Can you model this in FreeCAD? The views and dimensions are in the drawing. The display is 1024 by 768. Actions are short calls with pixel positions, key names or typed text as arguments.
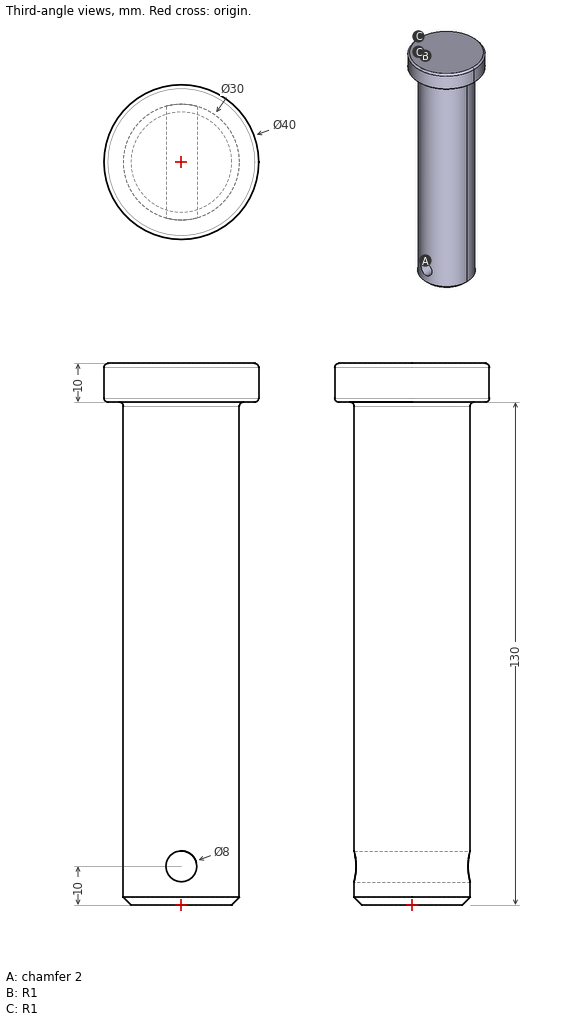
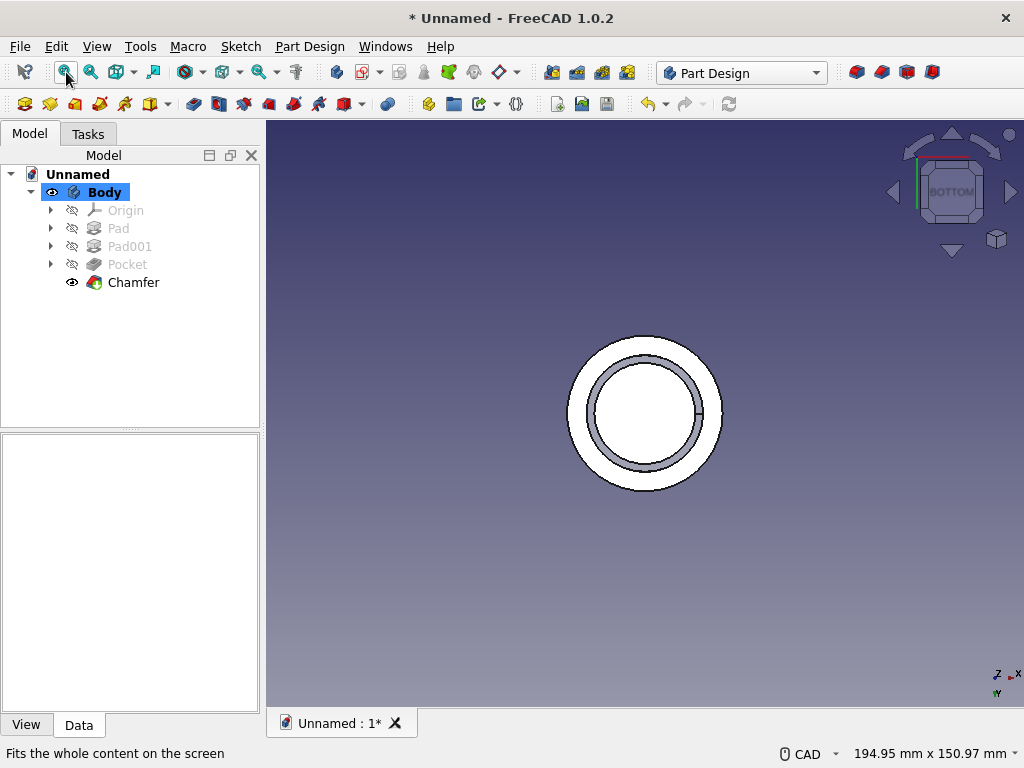
key(4)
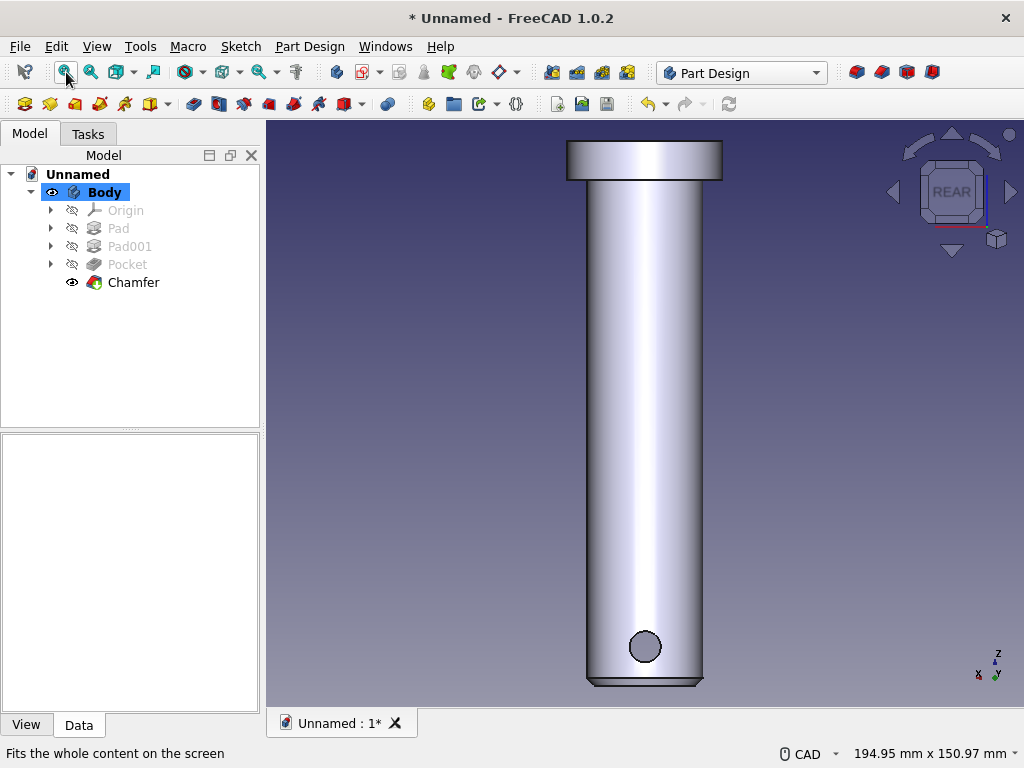
key(6)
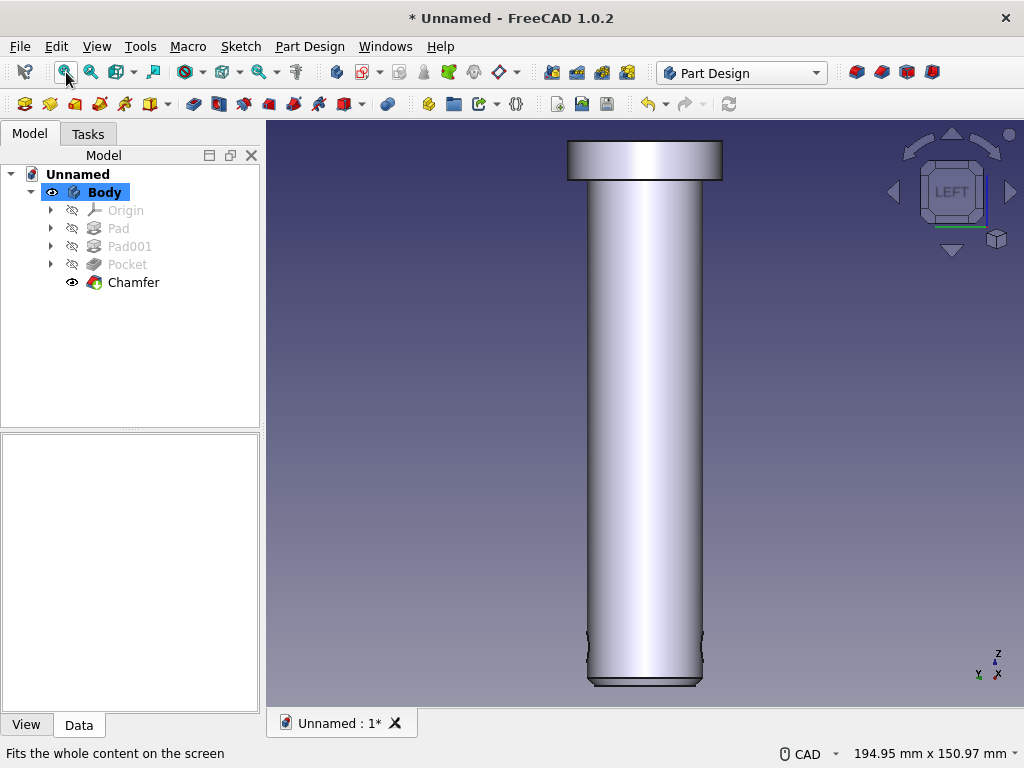
key(v)
key(3)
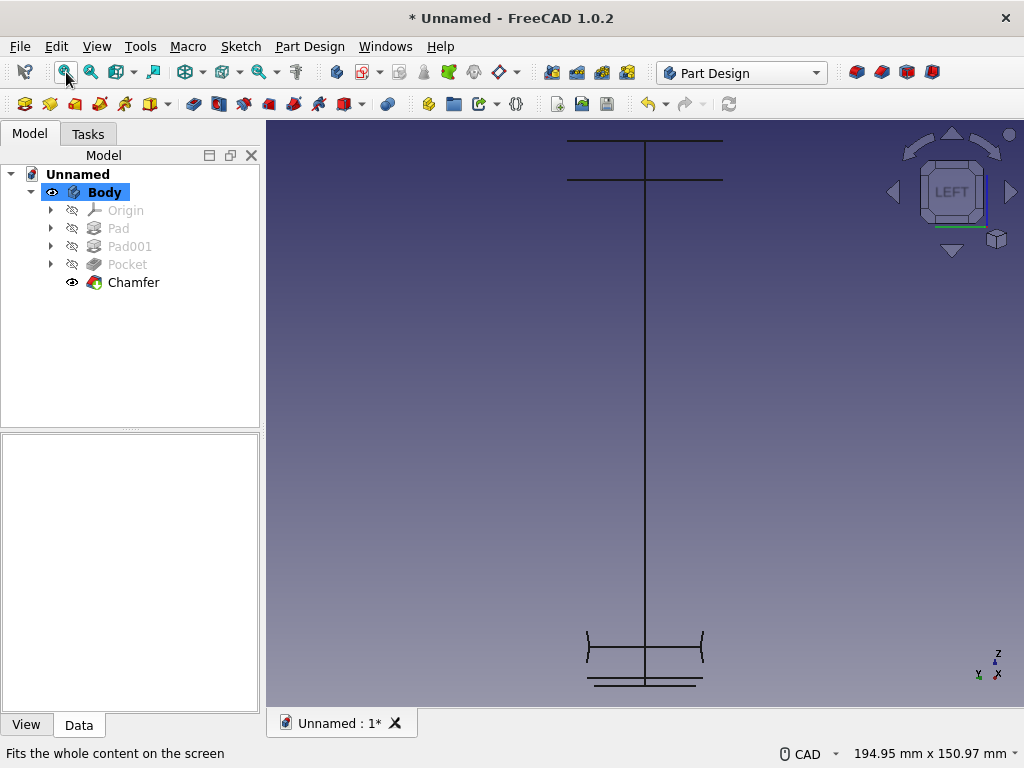
key(0)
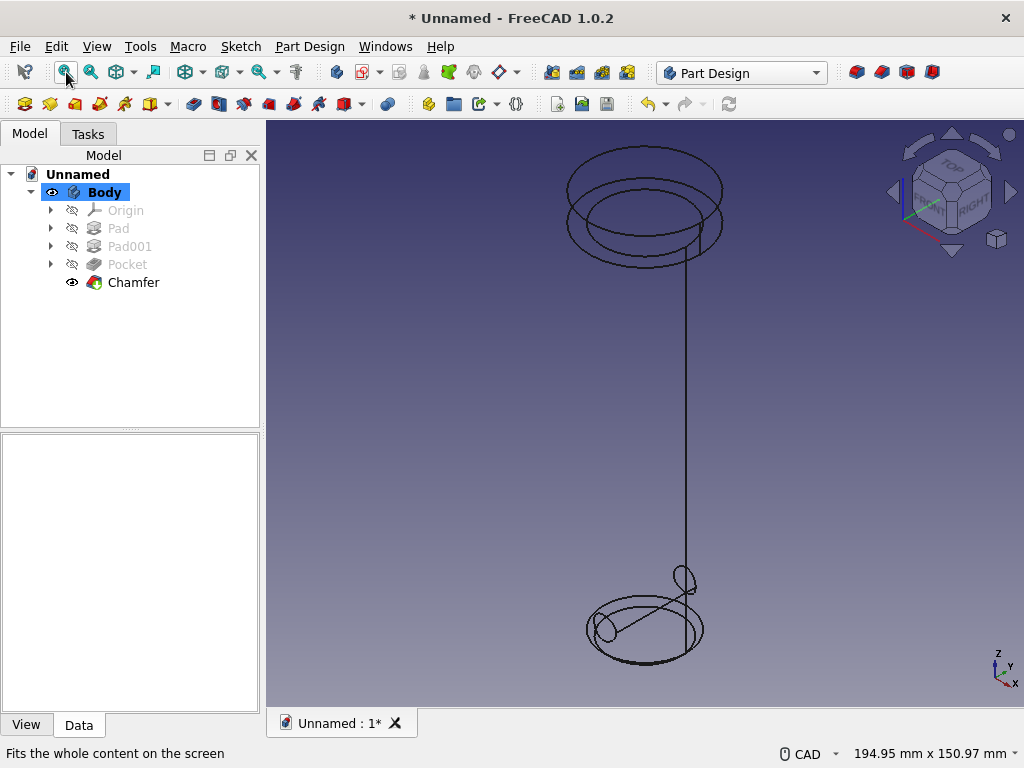
click(604, 198)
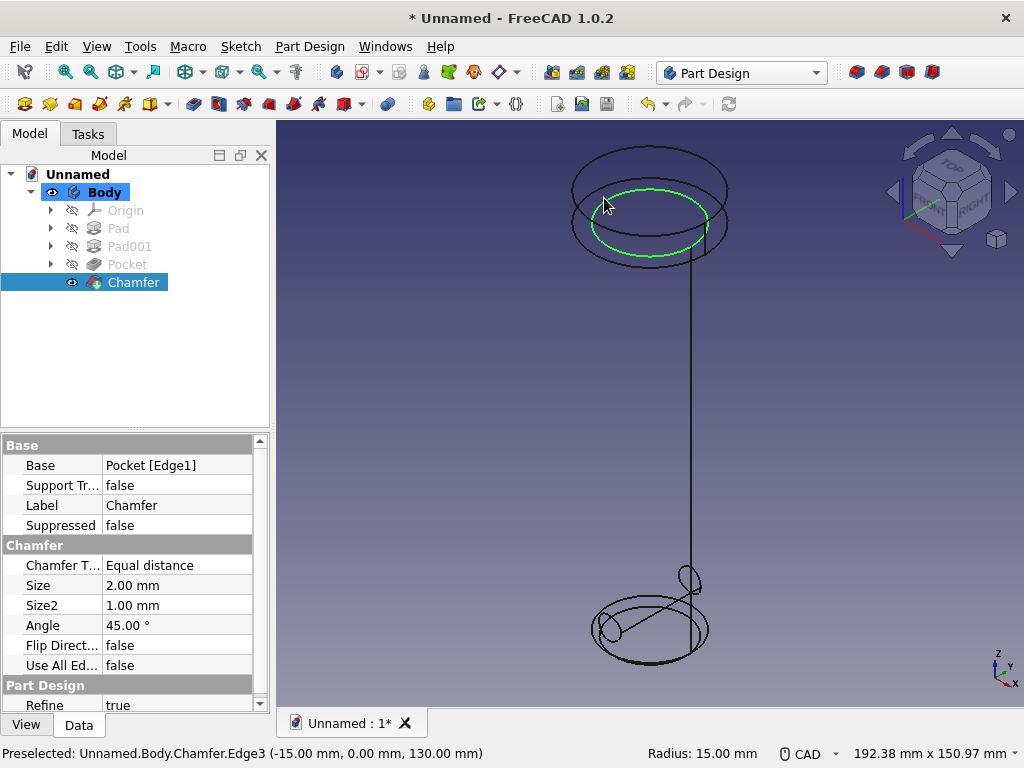
key(v)
key(1)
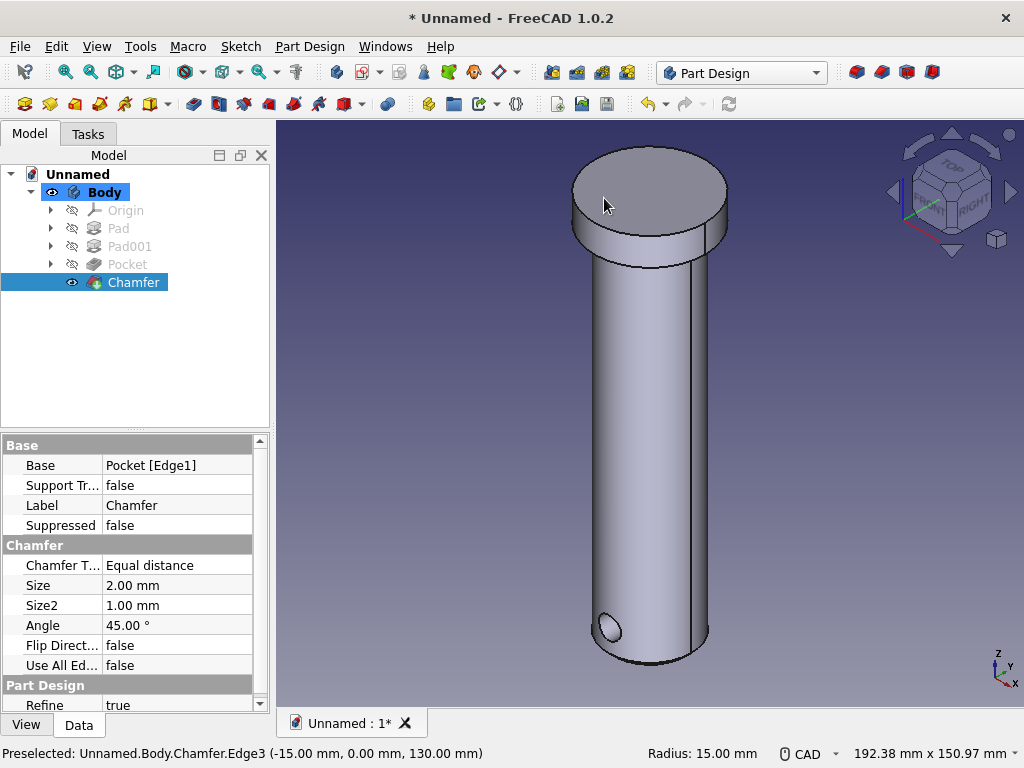
click(857, 72)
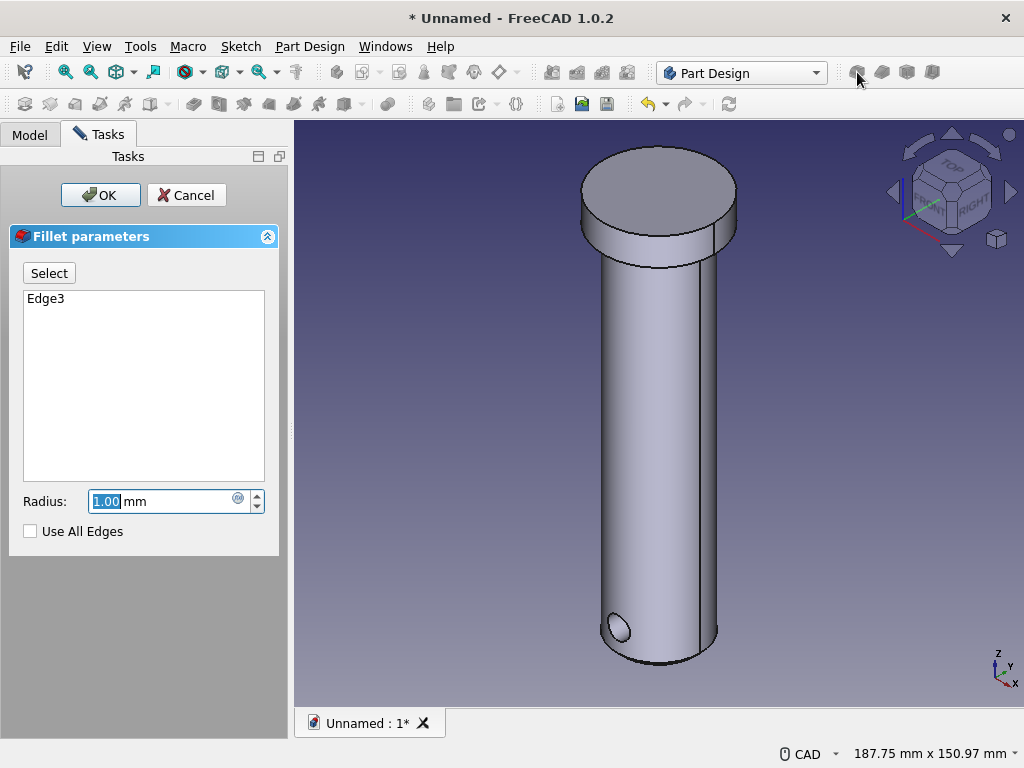
text(1)
key(Tab)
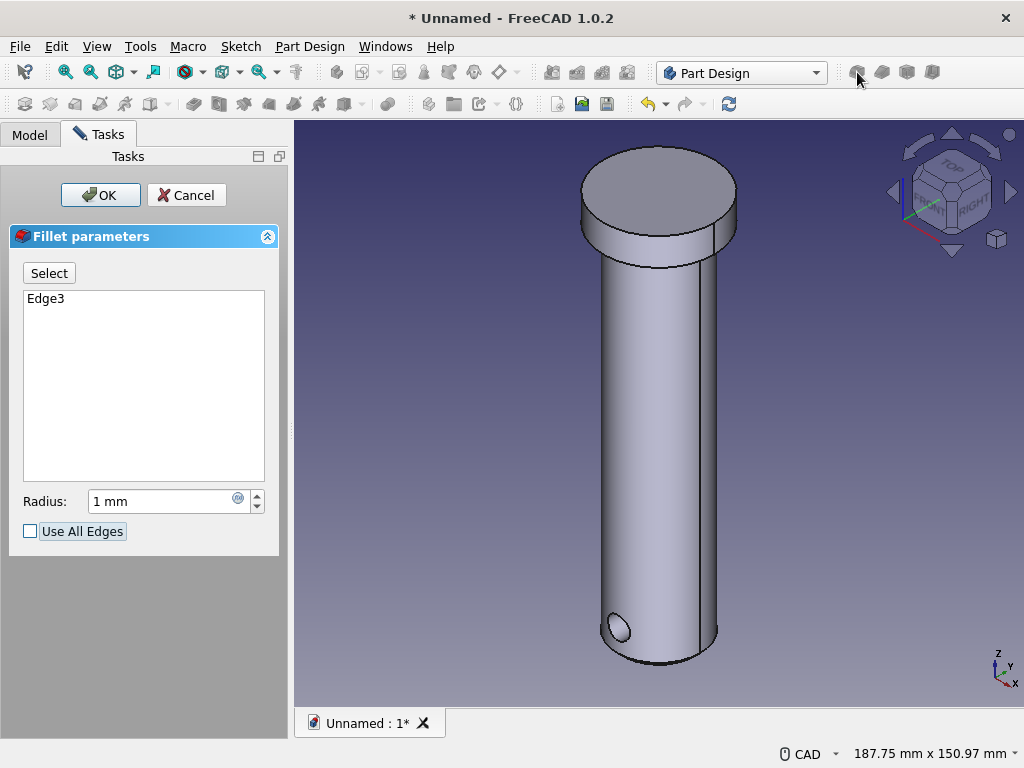
click(101, 195)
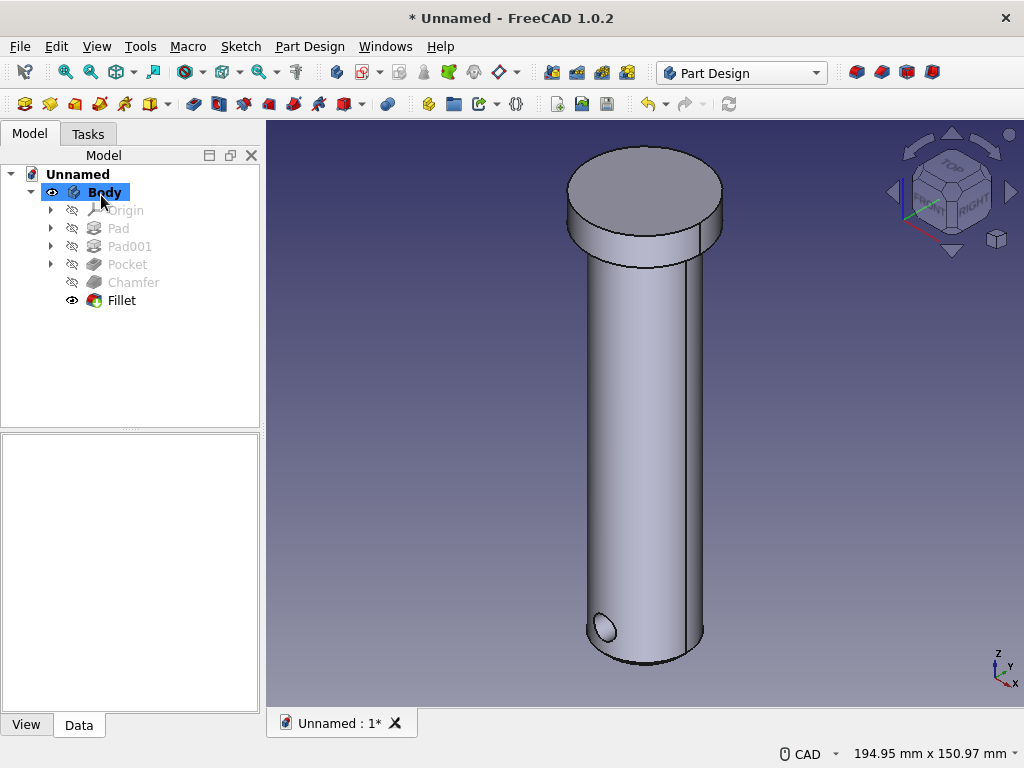
click(576, 211)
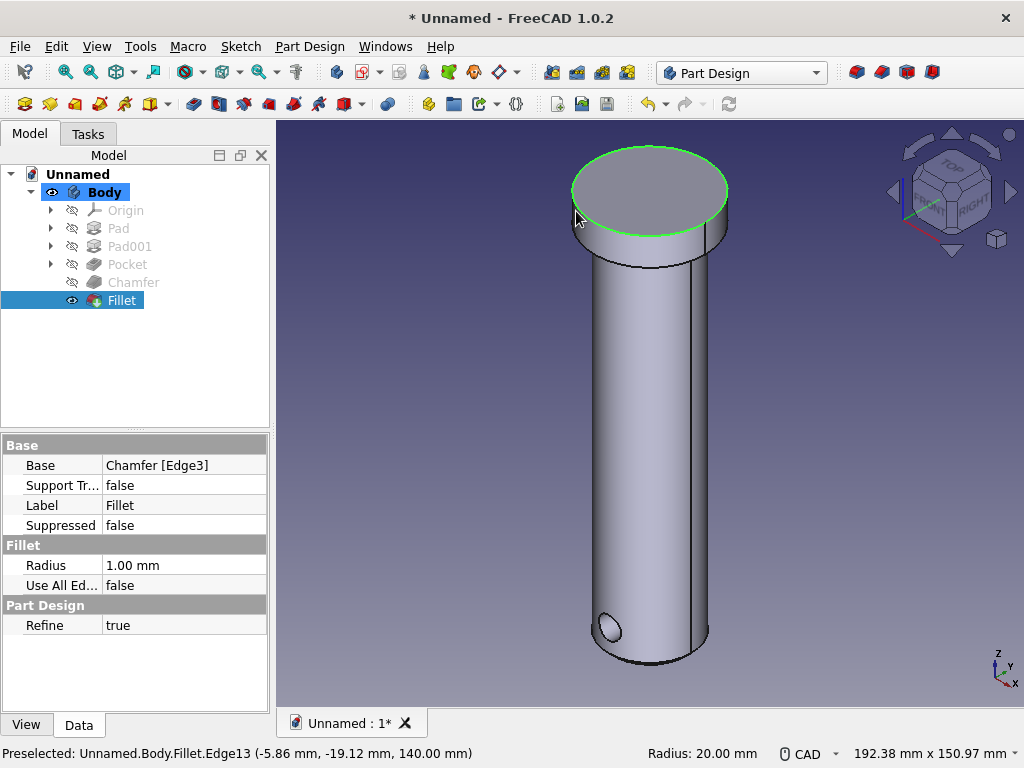
key(2)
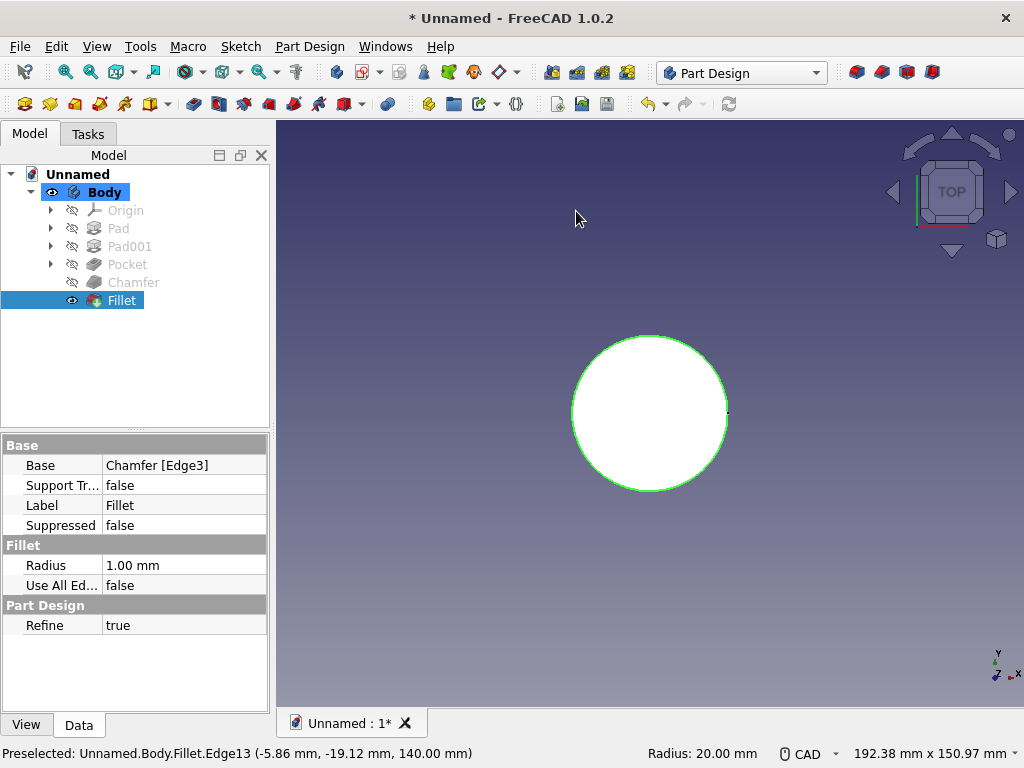
click(66, 72)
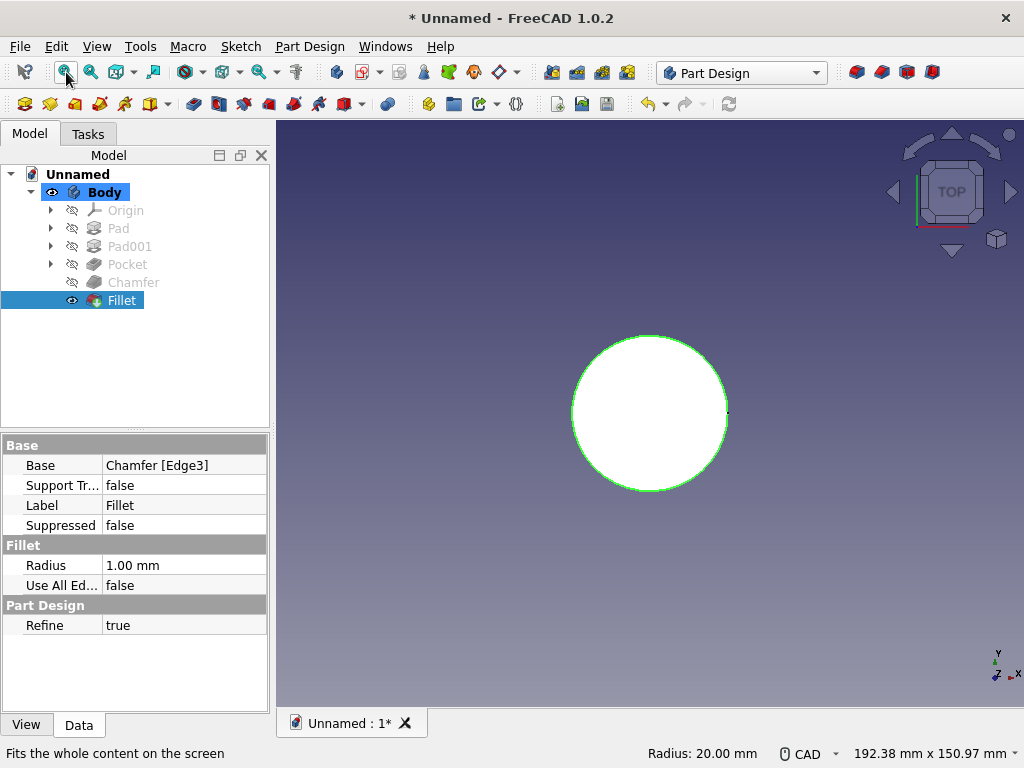
key(0)